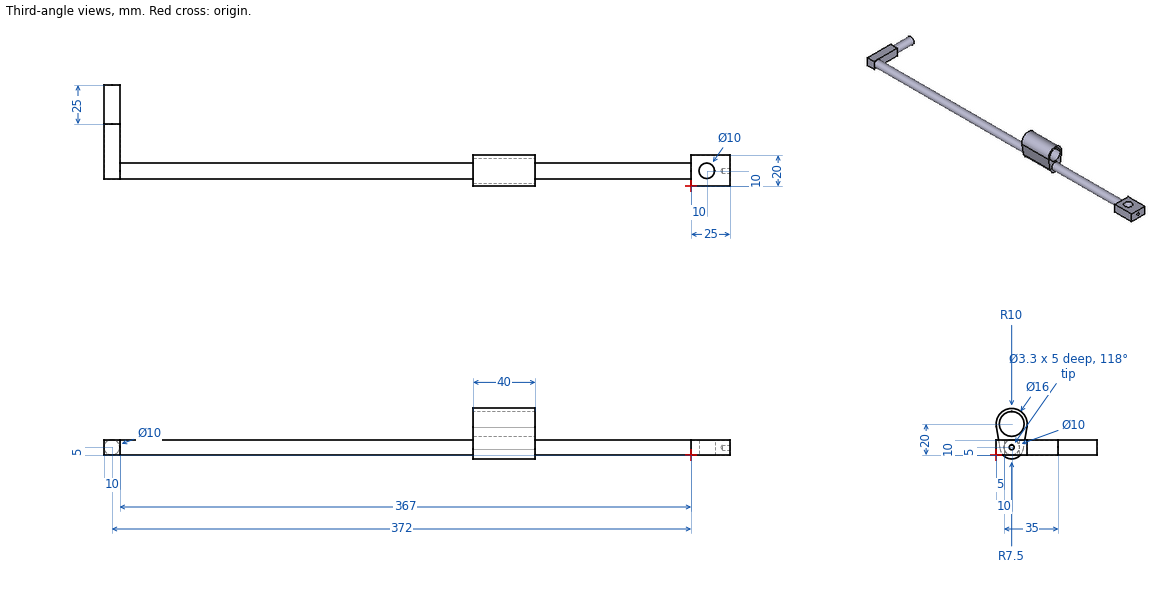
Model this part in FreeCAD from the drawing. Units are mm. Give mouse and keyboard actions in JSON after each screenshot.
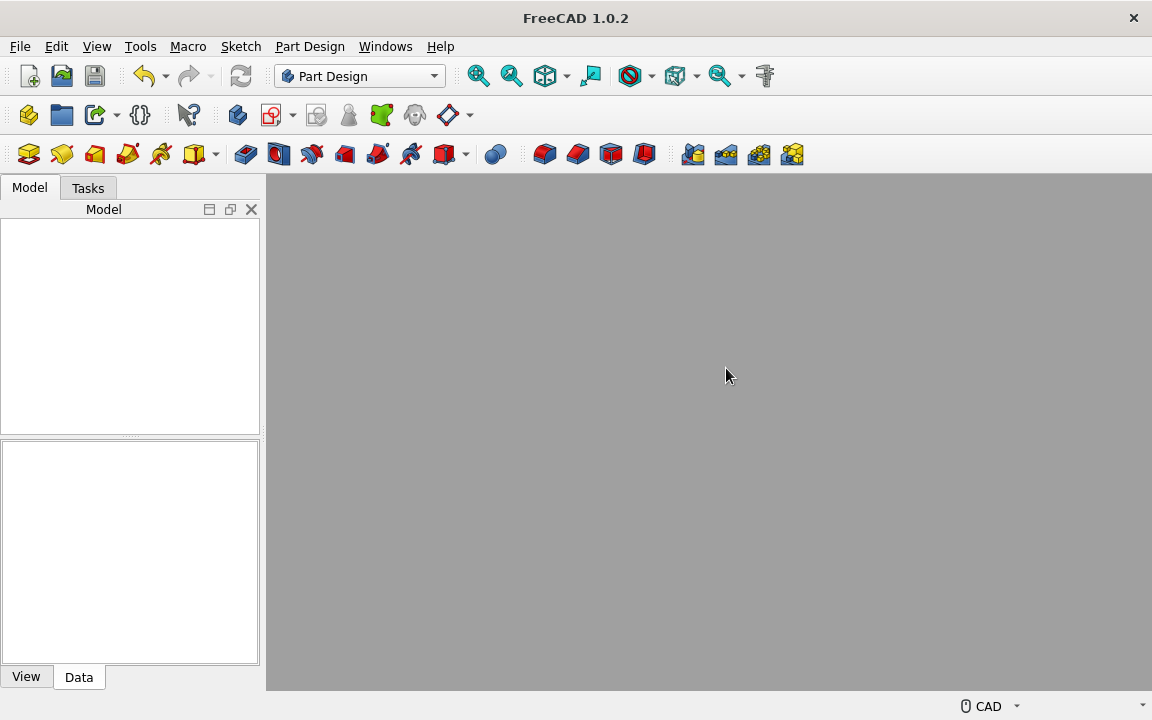
{"action": "left_click", "coordinate": [29, 76]}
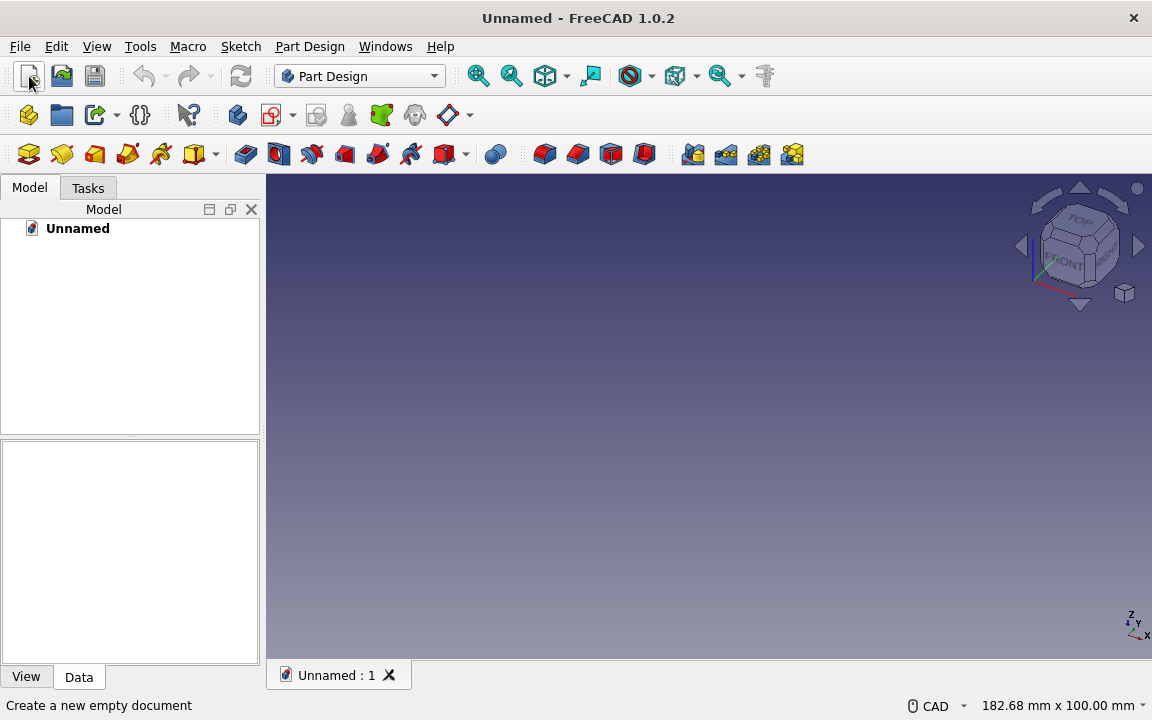
{"action": "left_click", "coordinate": [270, 116]}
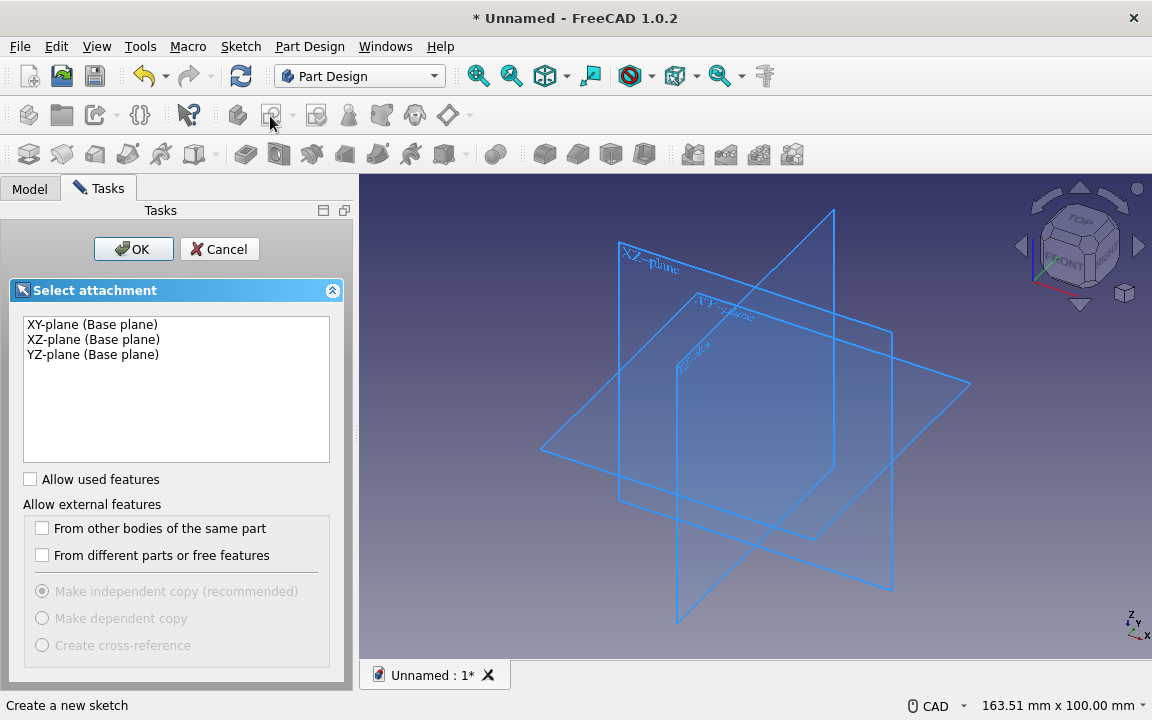
{"action": "left_click", "coordinate": [84, 324]}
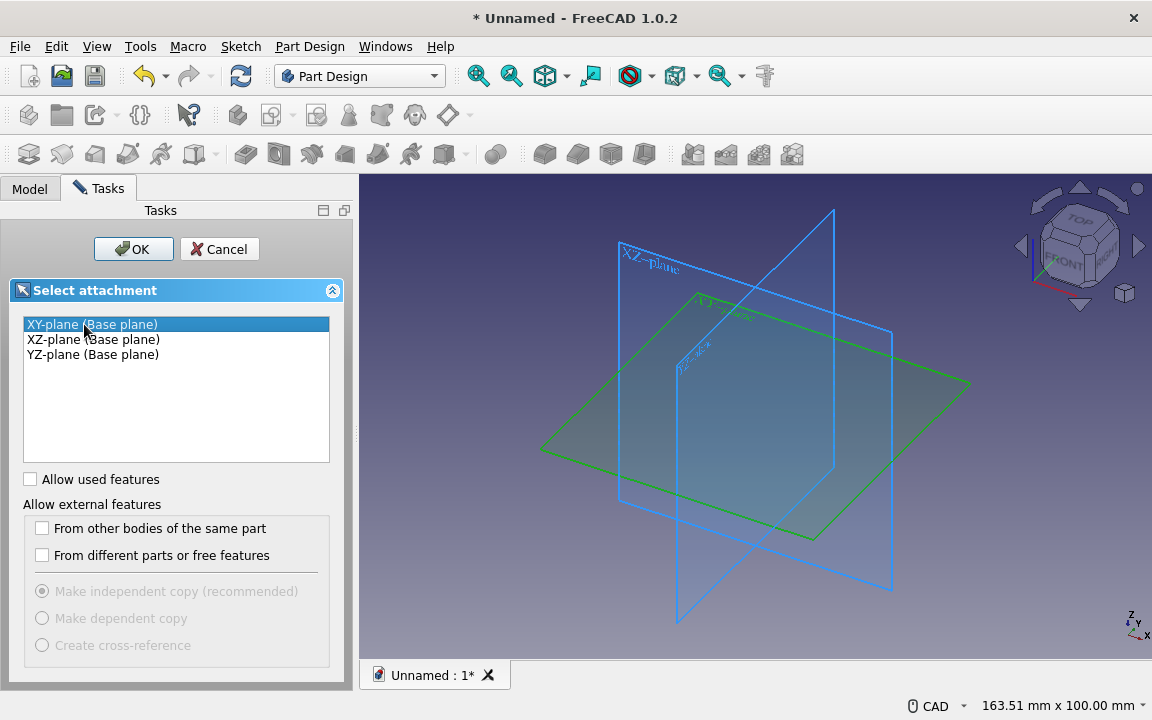
{"action": "left_click", "coordinate": [134, 249]}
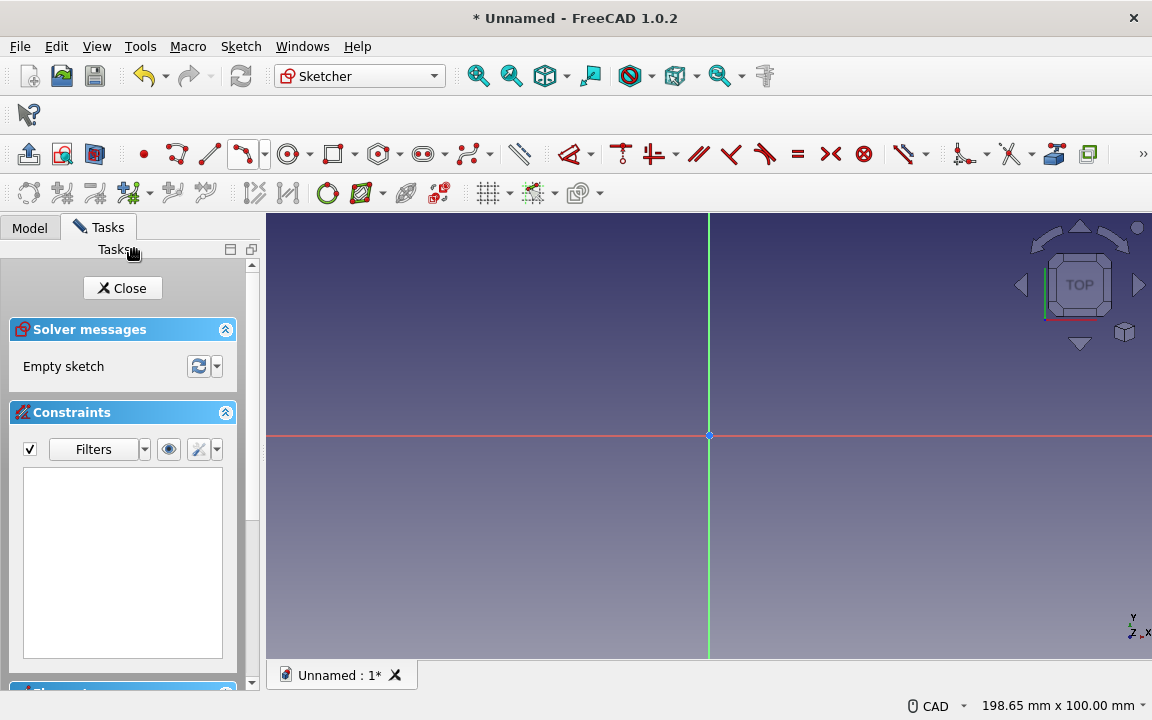
{"action": "scroll", "coordinate": [818, 372], "scroll_direction": "up", "scroll_amount": 6}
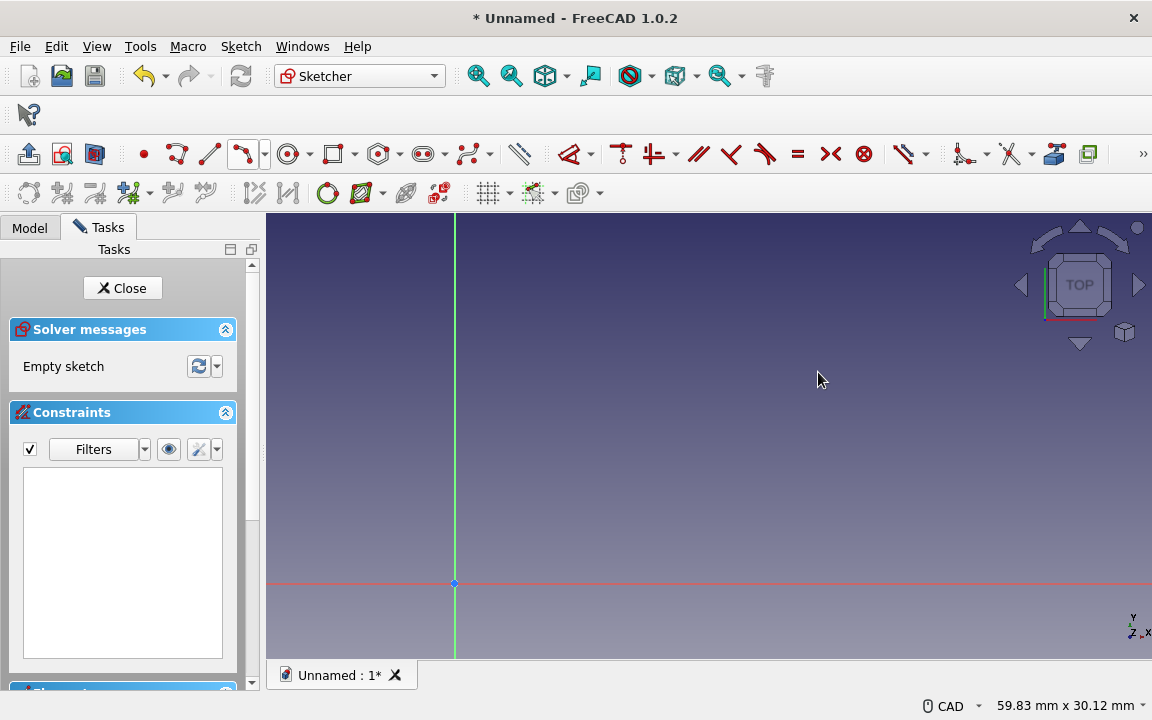
{"action": "key", "text": "g r"}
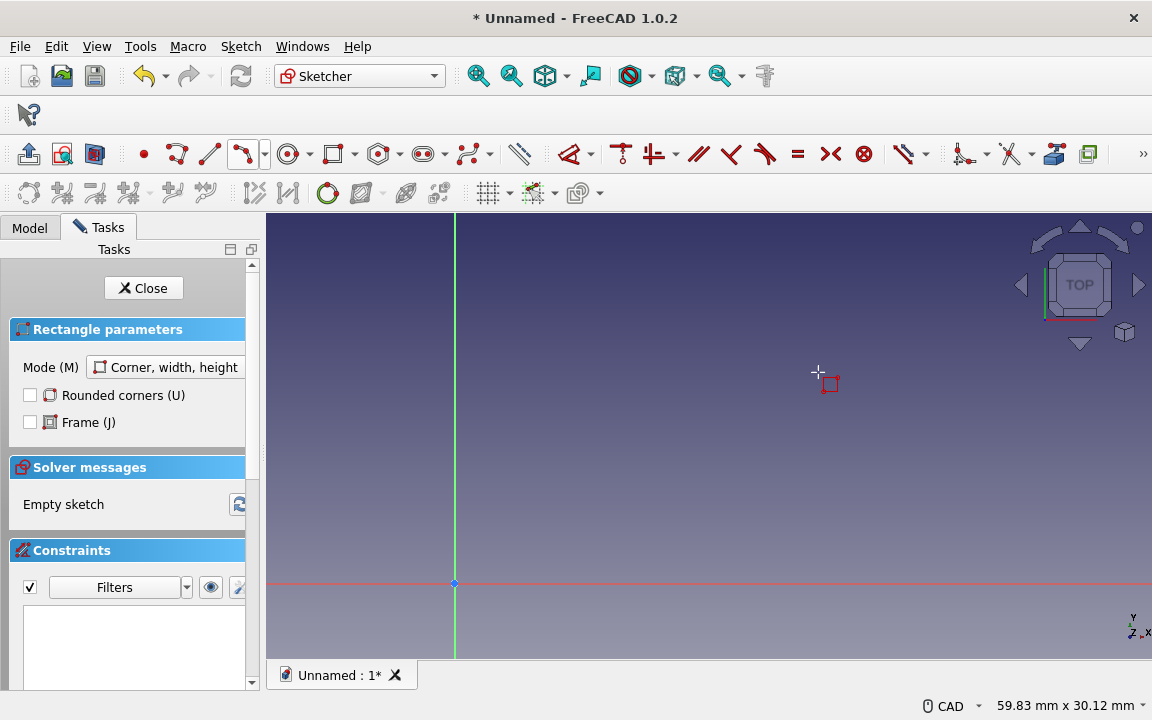
{"action": "left_click", "coordinate": [455, 584]}
{"action": "mouse_move", "coordinate": [825, 288]}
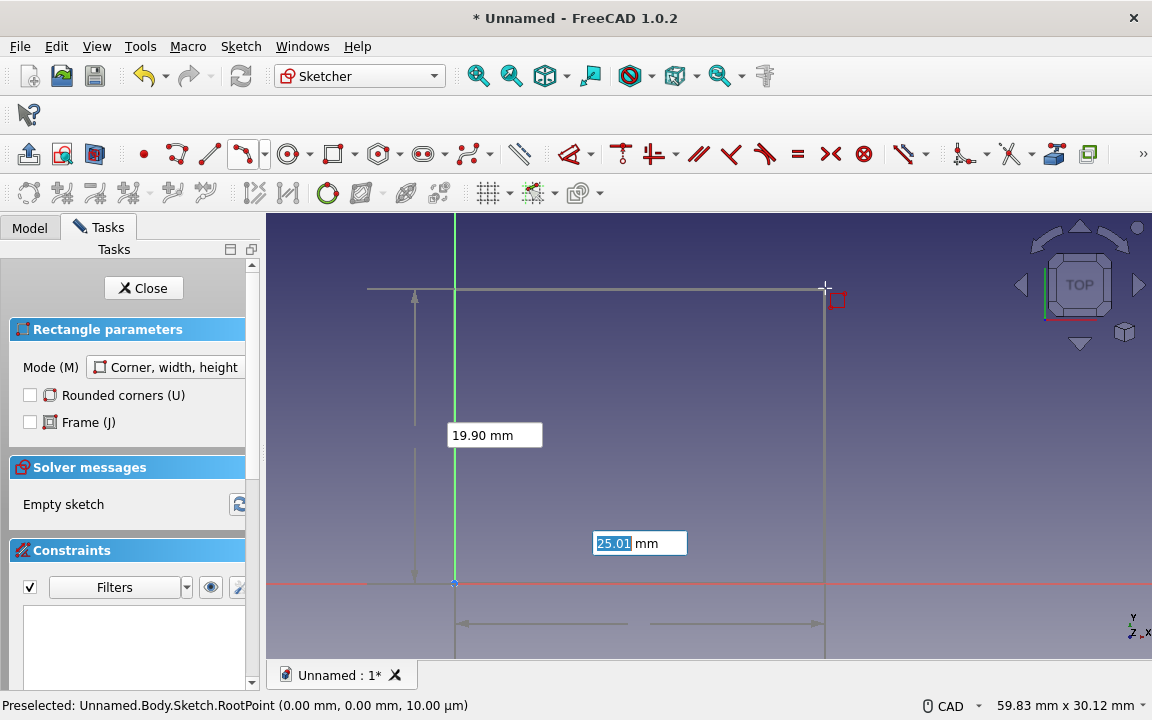
{"action": "type", "text": "25"}
{"action": "key", "text": "Tab"}
{"action": "type", "text": "20"}
{"action": "key", "text": "Return"}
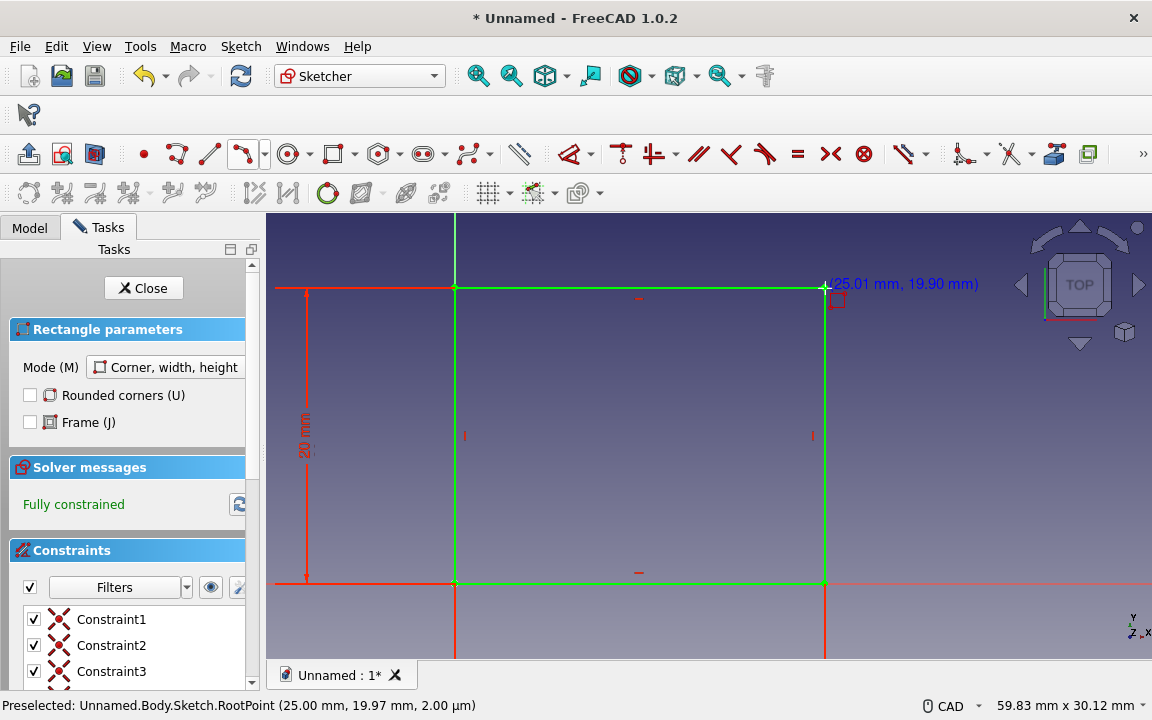
{"action": "key", "text": "g c"}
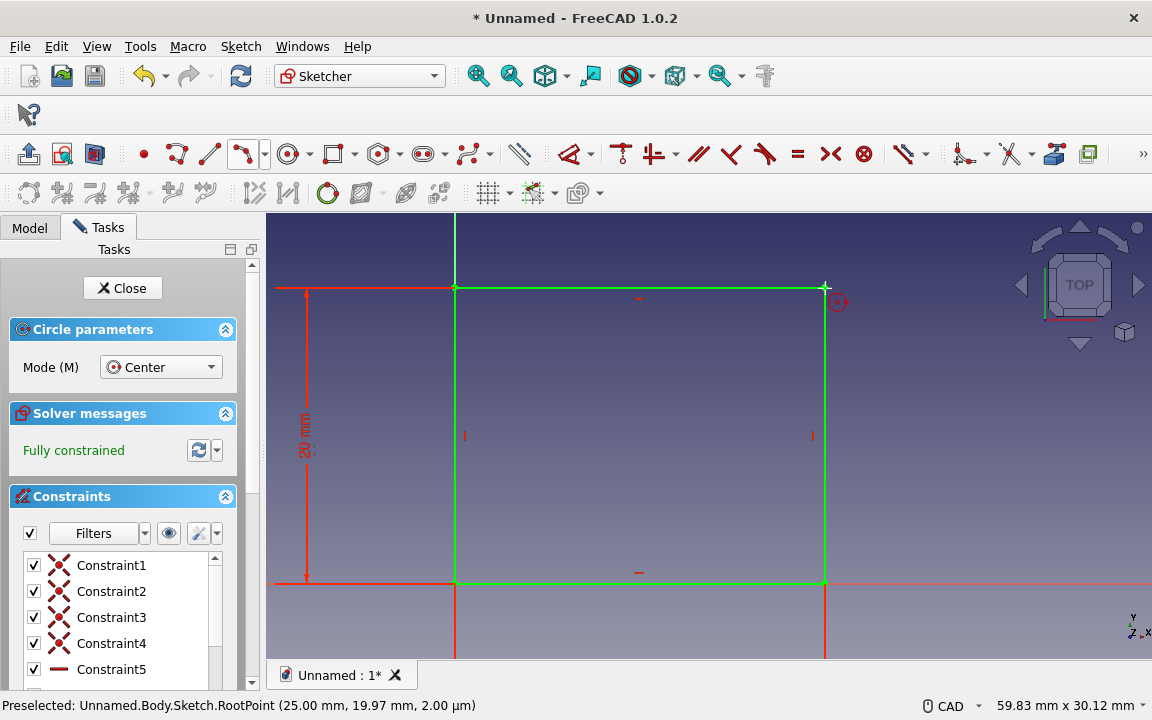
{"action": "left_click", "coordinate": [603, 436]}
{"action": "mouse_move", "coordinate": [655, 383]}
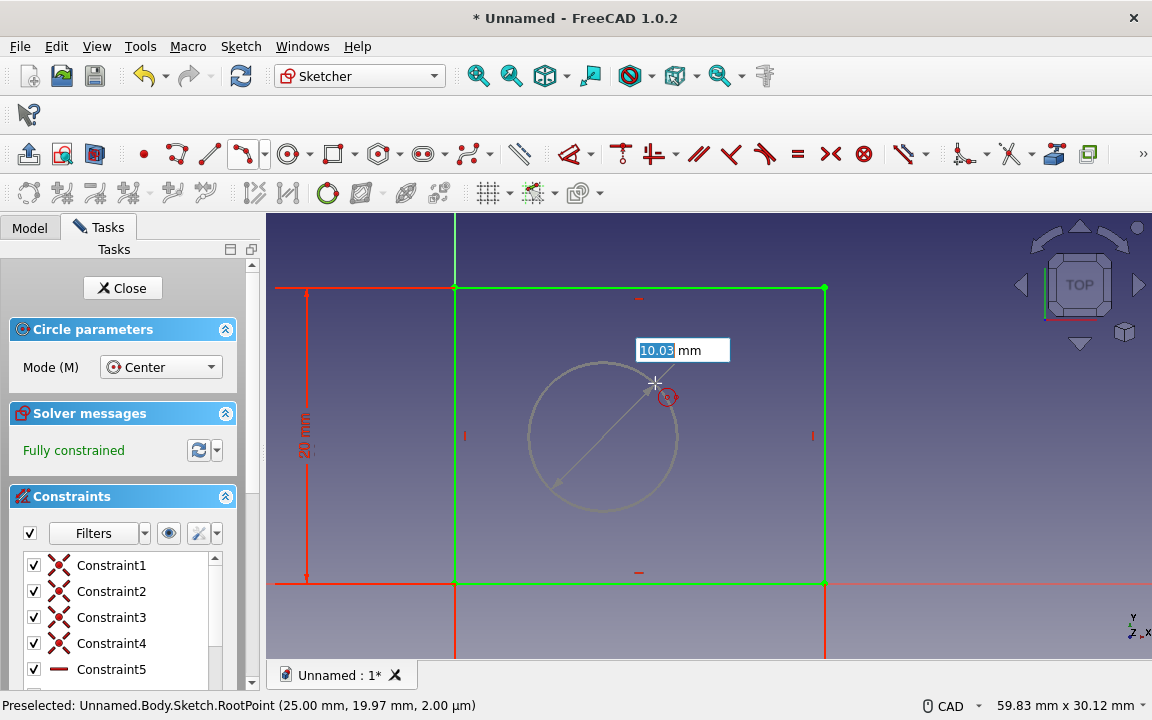
{"action": "type", "text": "10"}
{"action": "key", "text": "Return"}
{"action": "key", "text": "Escape"}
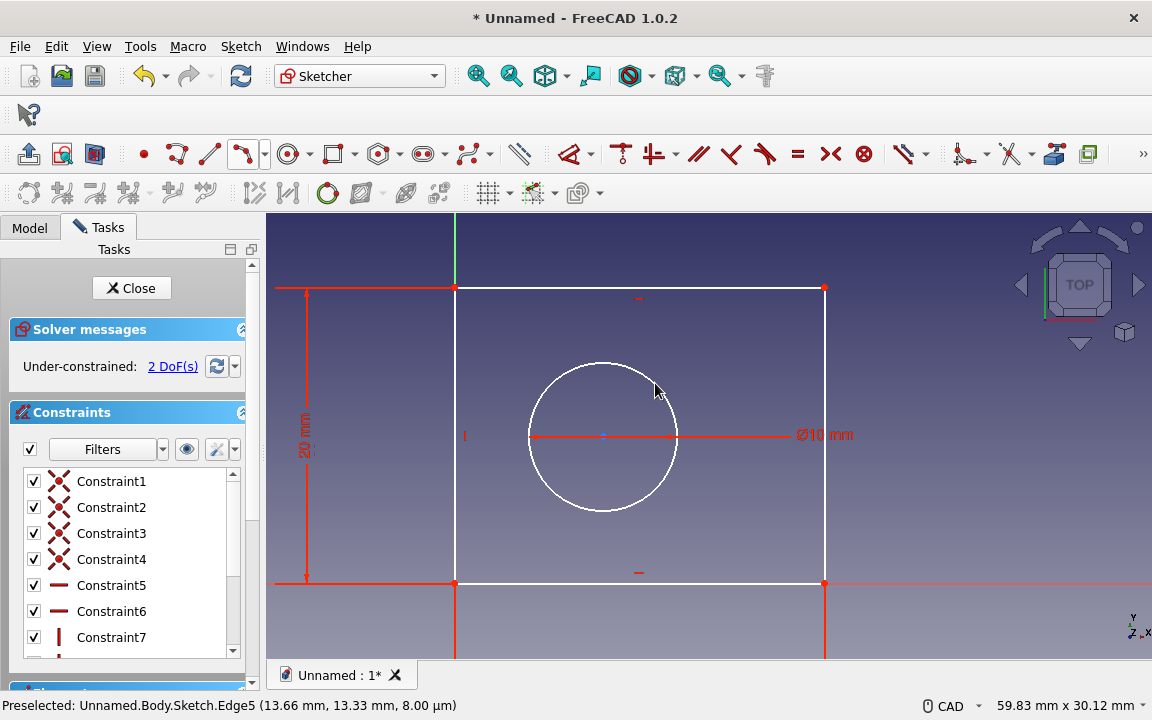
{"action": "left_click", "coordinate": [568, 154]}